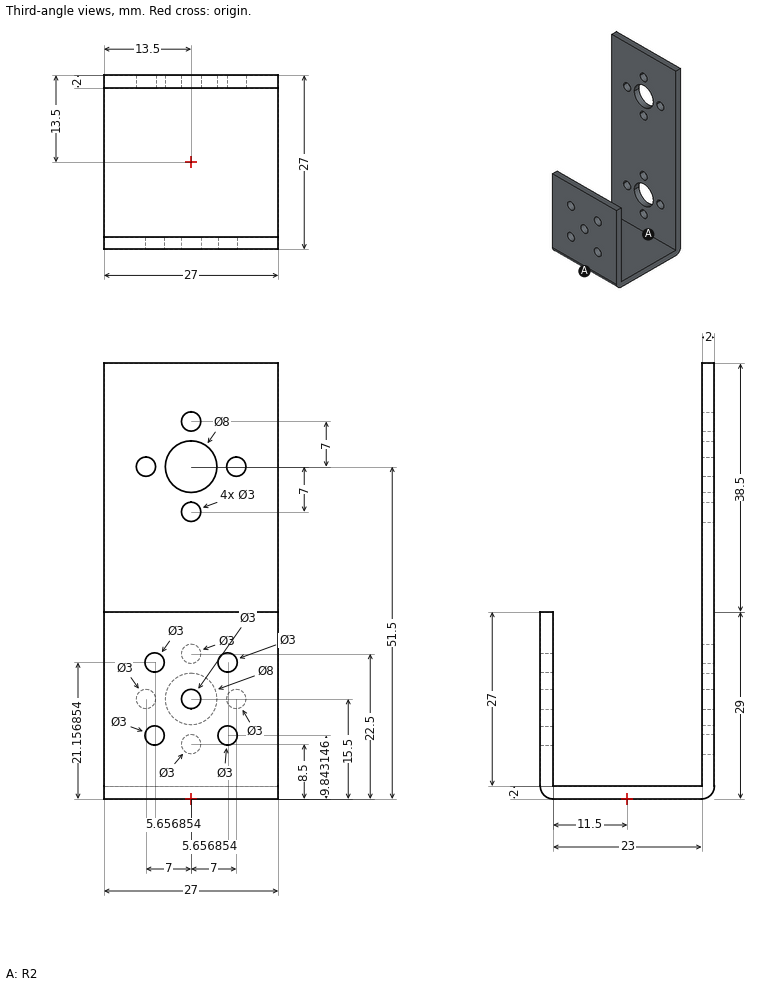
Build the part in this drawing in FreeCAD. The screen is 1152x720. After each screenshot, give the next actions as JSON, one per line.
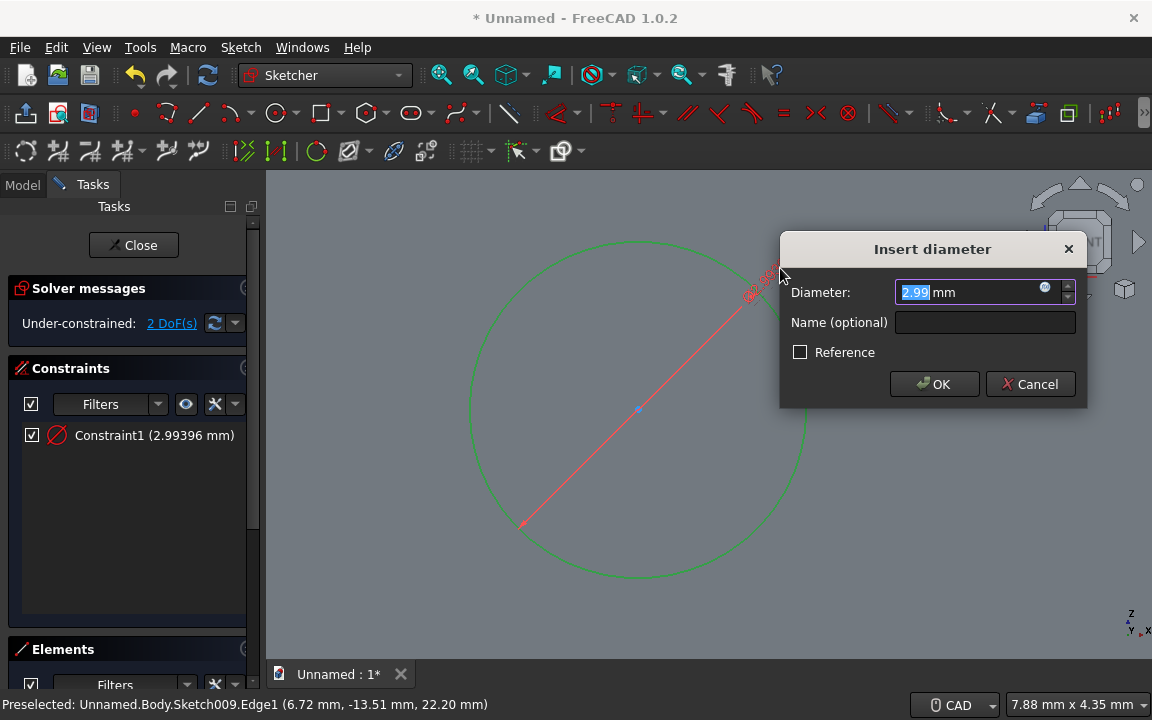
{"action": "type", "text": "3"}
{"action": "key", "text": "Return"}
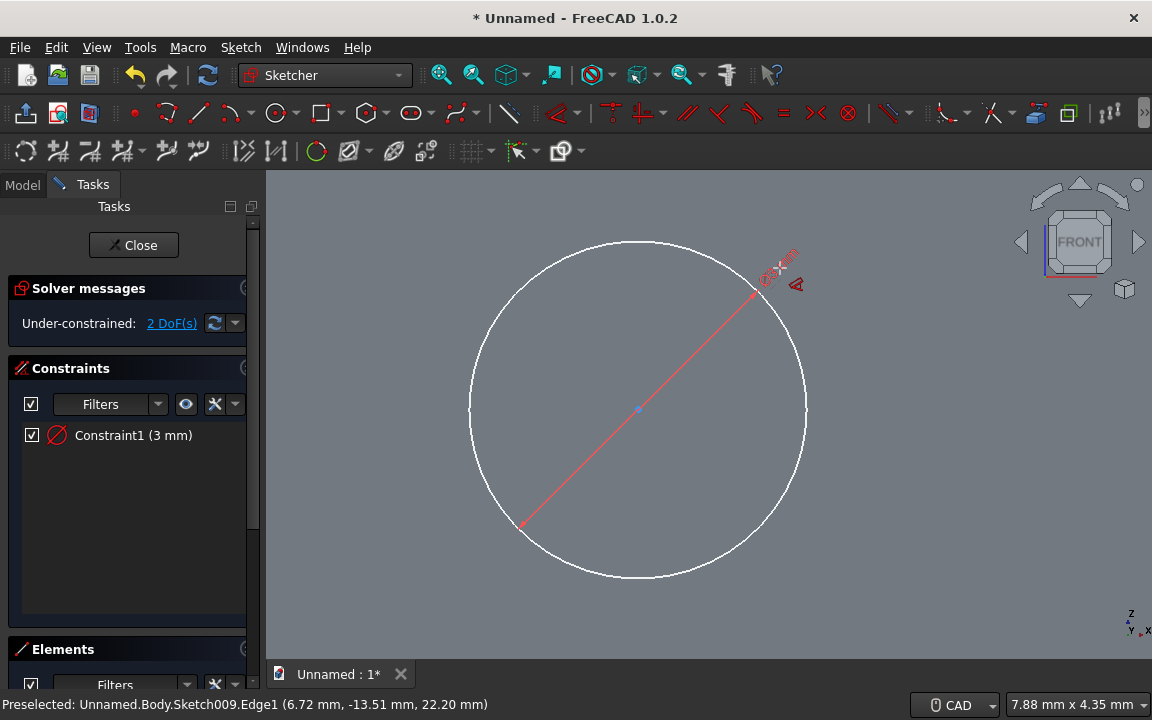
{"action": "left_click", "coordinate": [638, 410]}
{"action": "left_click", "coordinate": [387, 376]}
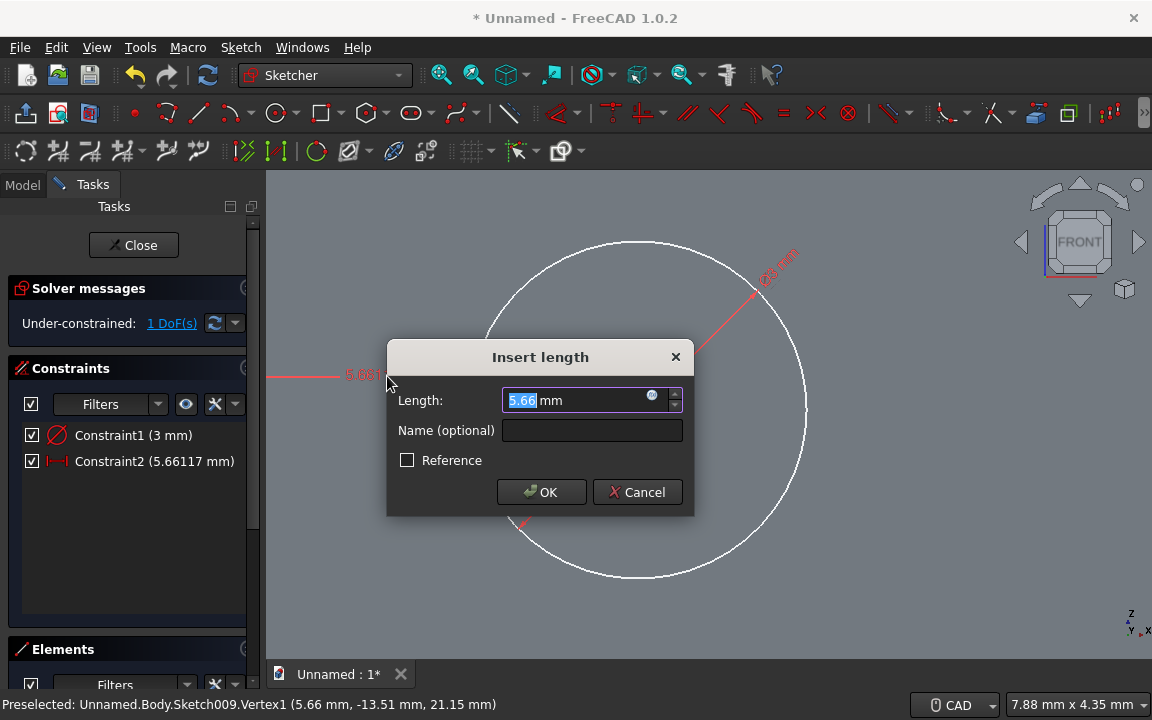
{"action": "type", "text": "5.656854"}
{"action": "key", "text": "Return"}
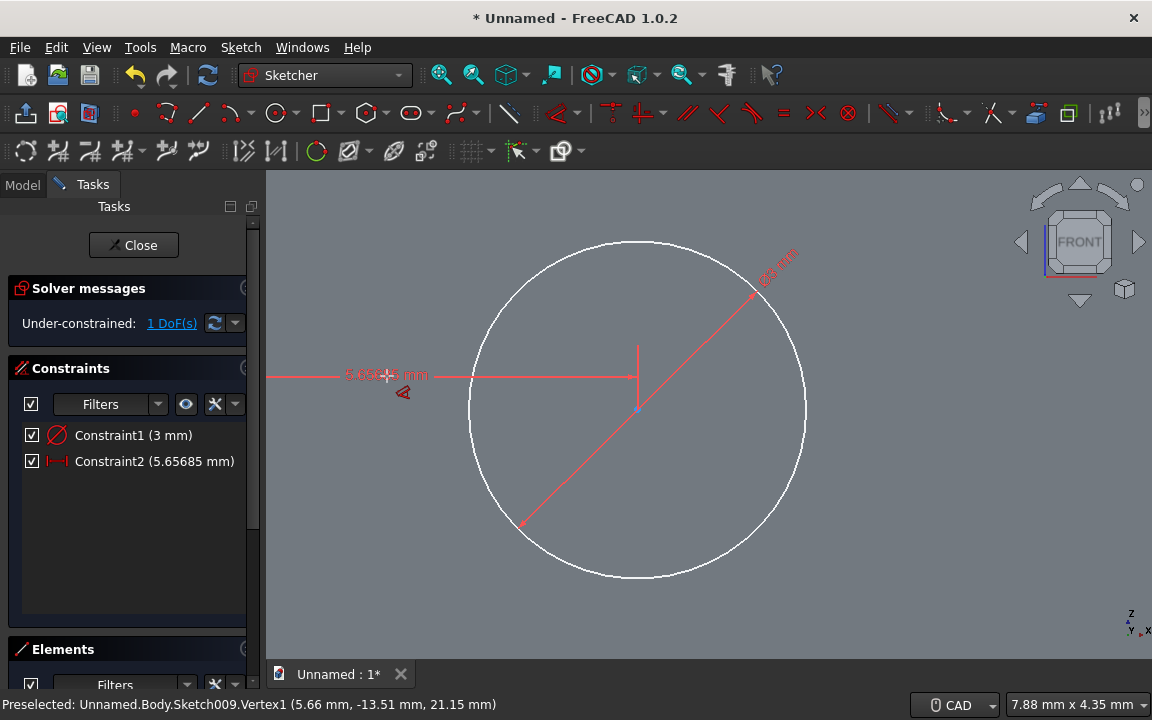
{"action": "left_click", "coordinate": [638, 410]}
{"action": "left_click", "coordinate": [672, 521]}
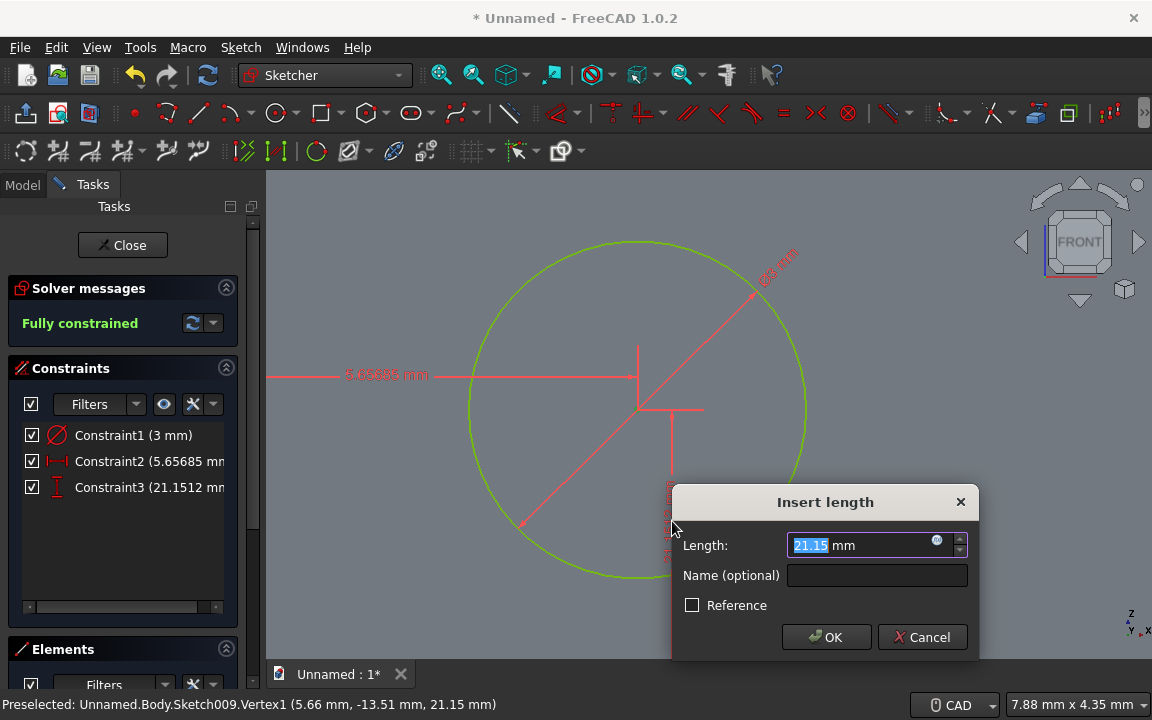
{"action": "type", "text": "21.156854"}
{"action": "key", "text": "Return"}
{"action": "key", "text": "Escape"}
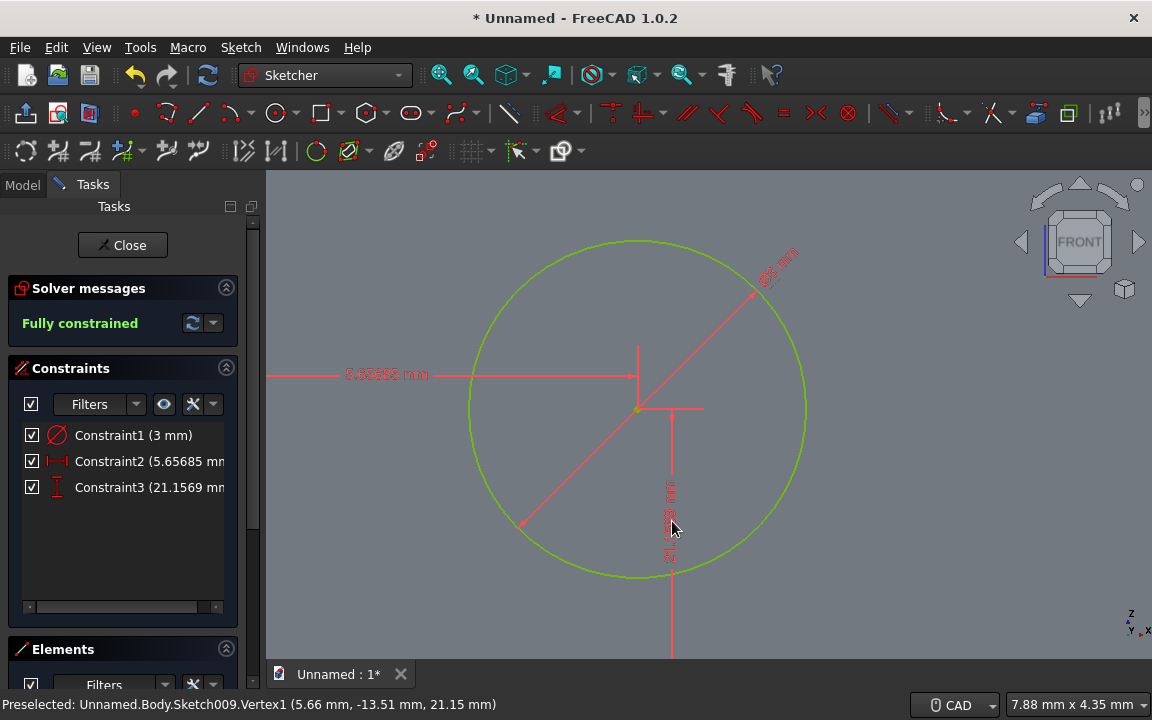
{"action": "left_click", "coordinate": [123, 245]}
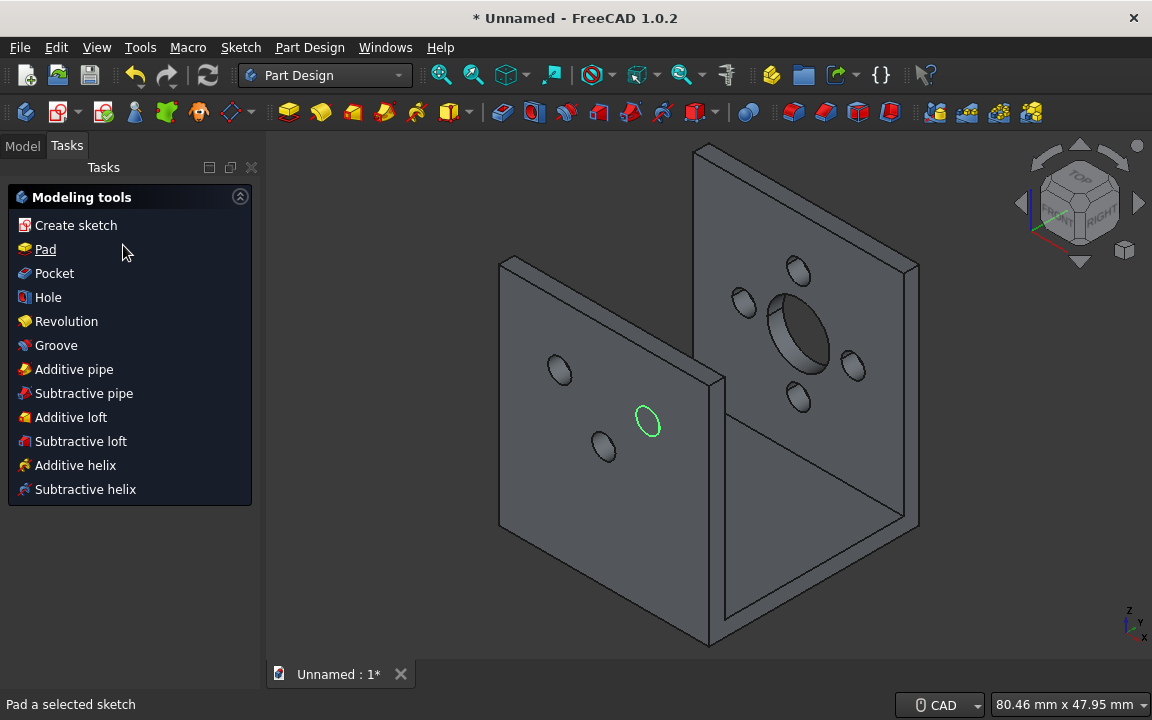
{"action": "left_click", "coordinate": [504, 112]}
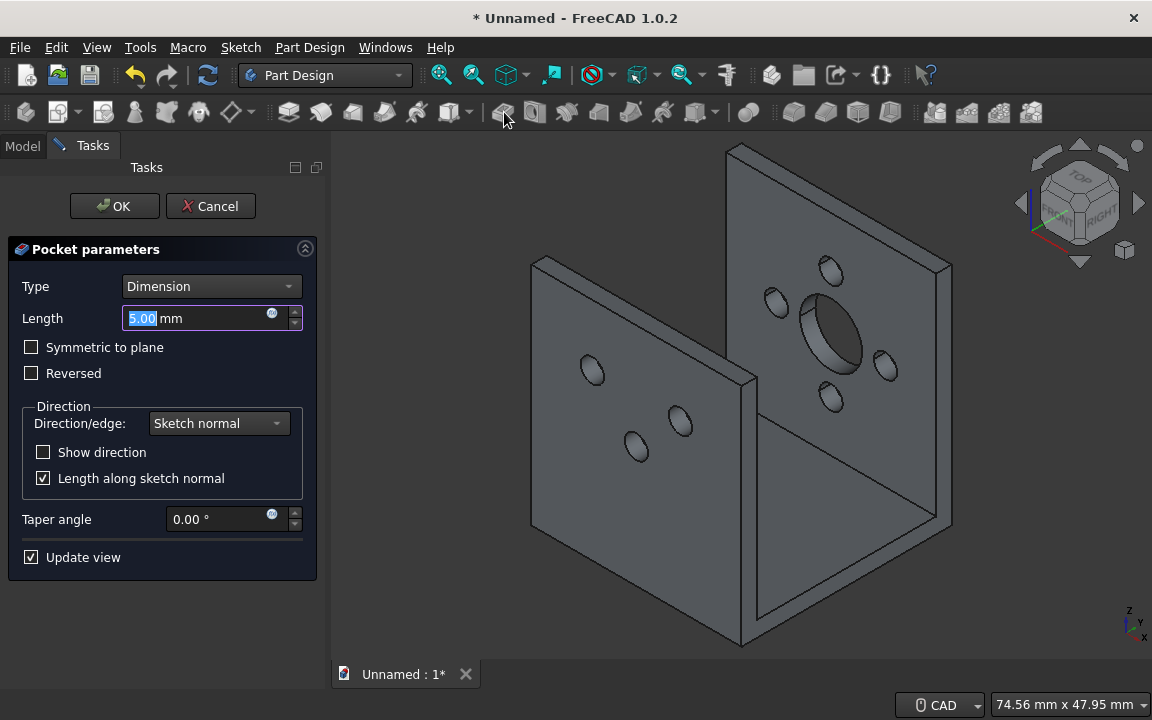
{"action": "left_click", "coordinate": [212, 286]}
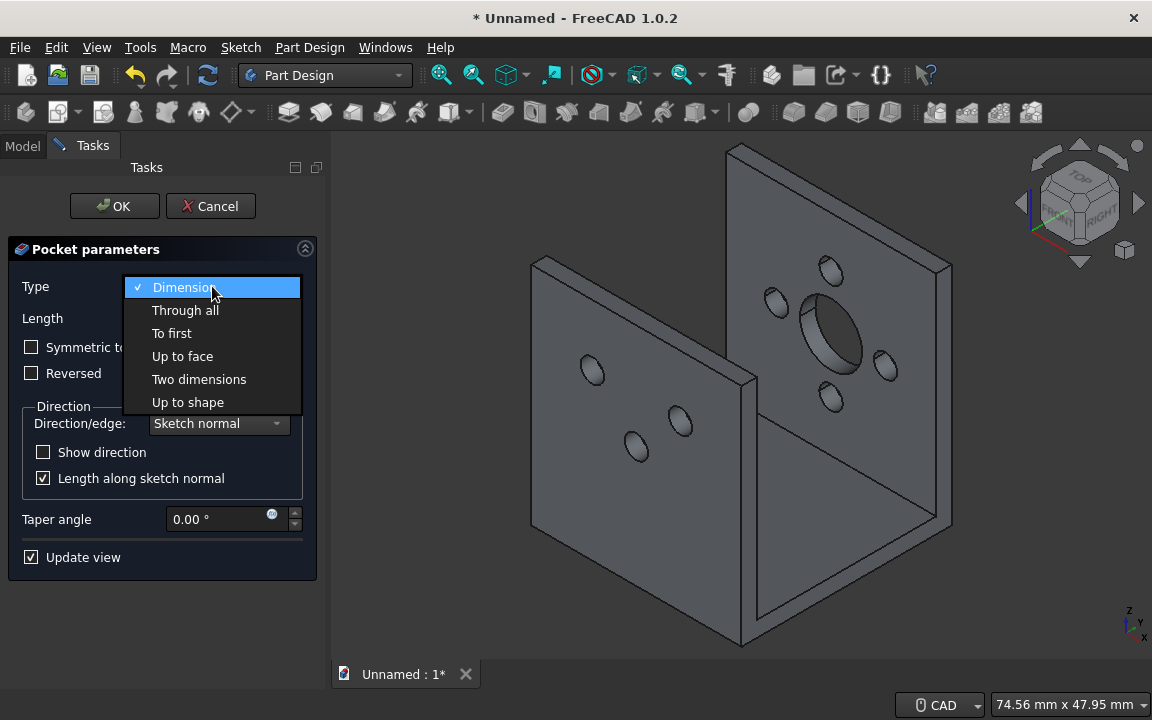
{"action": "left_click", "coordinate": [212, 334]}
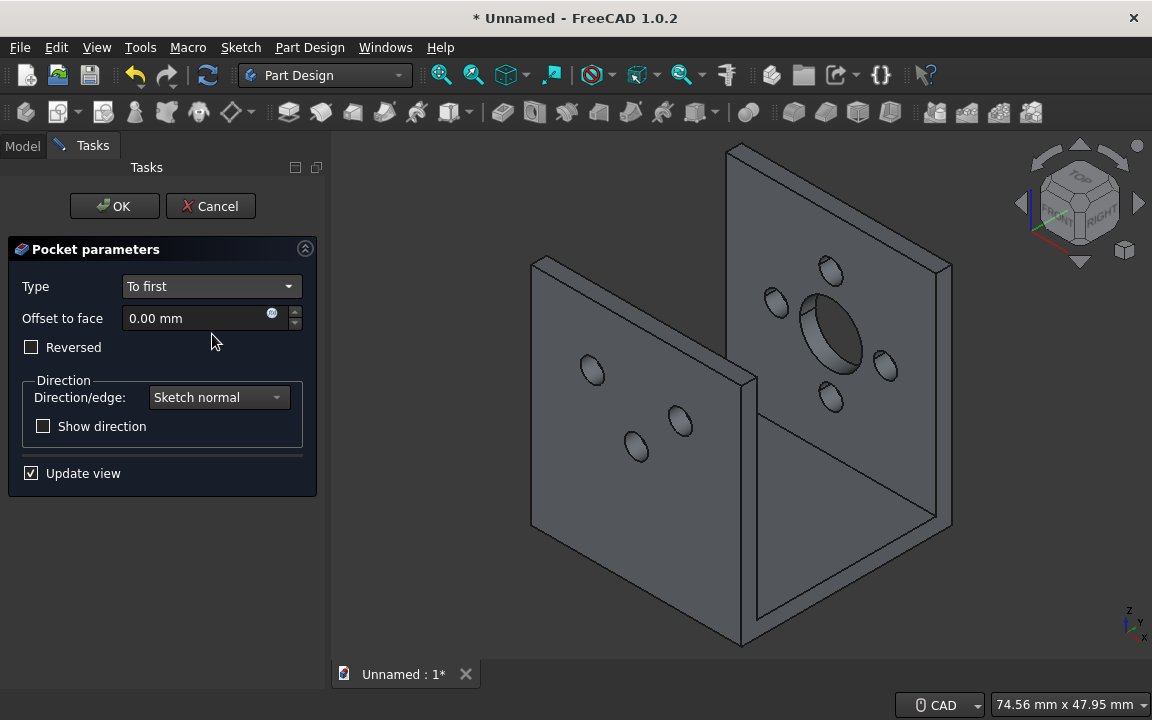
{"action": "left_click", "coordinate": [115, 206]}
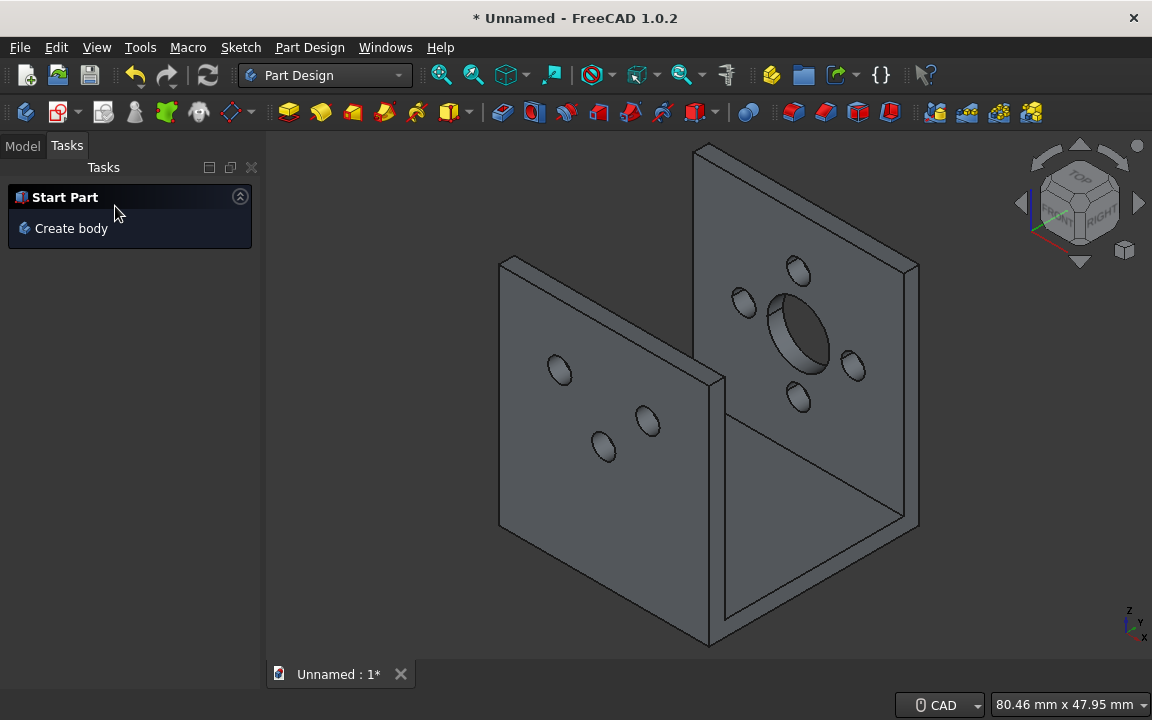
{"action": "left_click", "coordinate": [634, 547]}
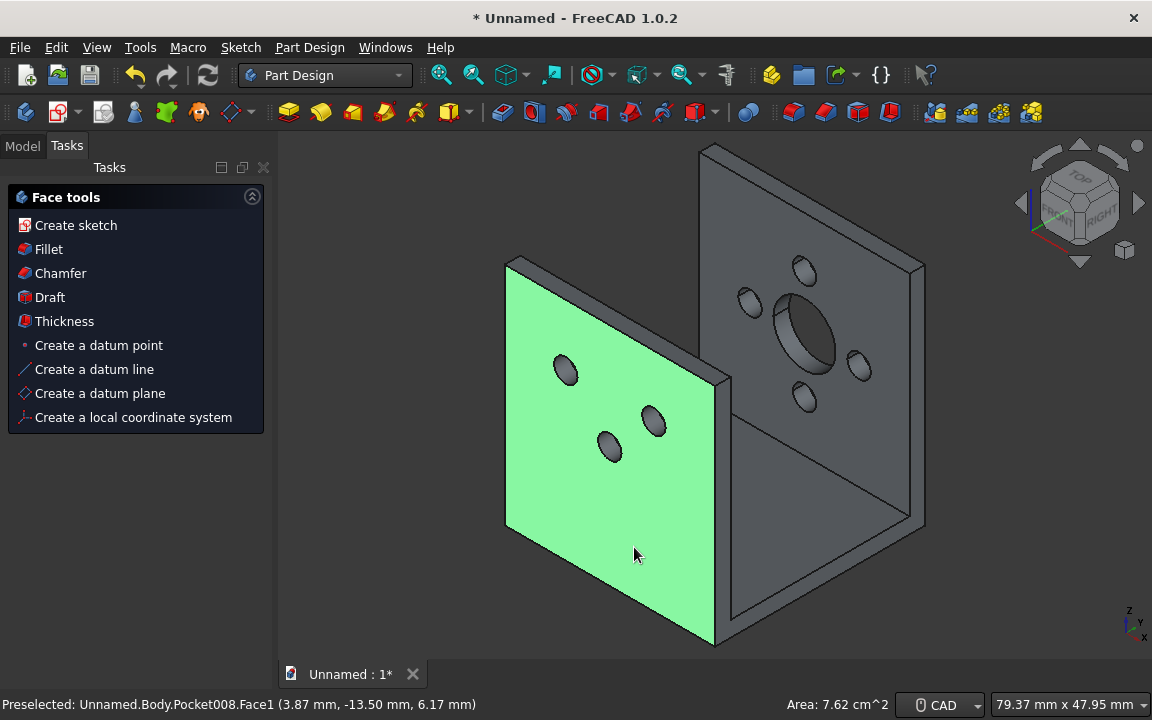
{"action": "left_click", "coordinate": [58, 112]}